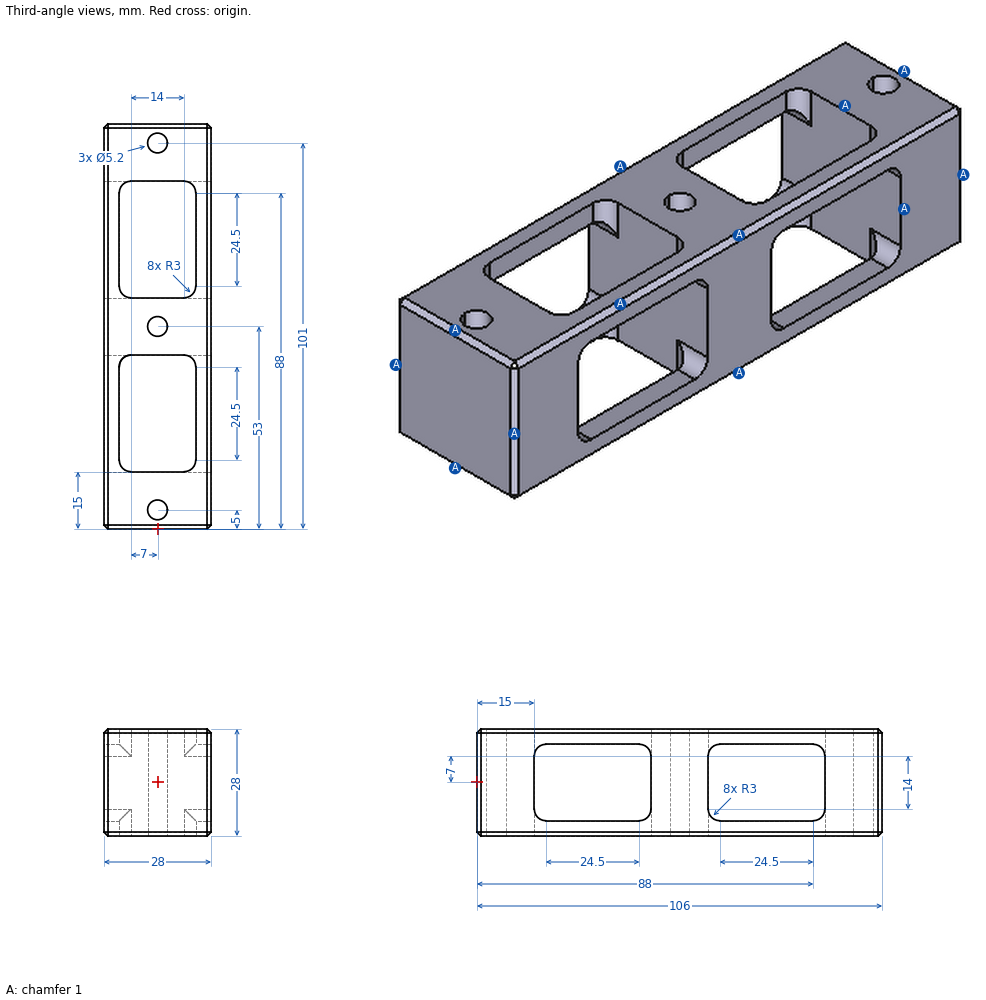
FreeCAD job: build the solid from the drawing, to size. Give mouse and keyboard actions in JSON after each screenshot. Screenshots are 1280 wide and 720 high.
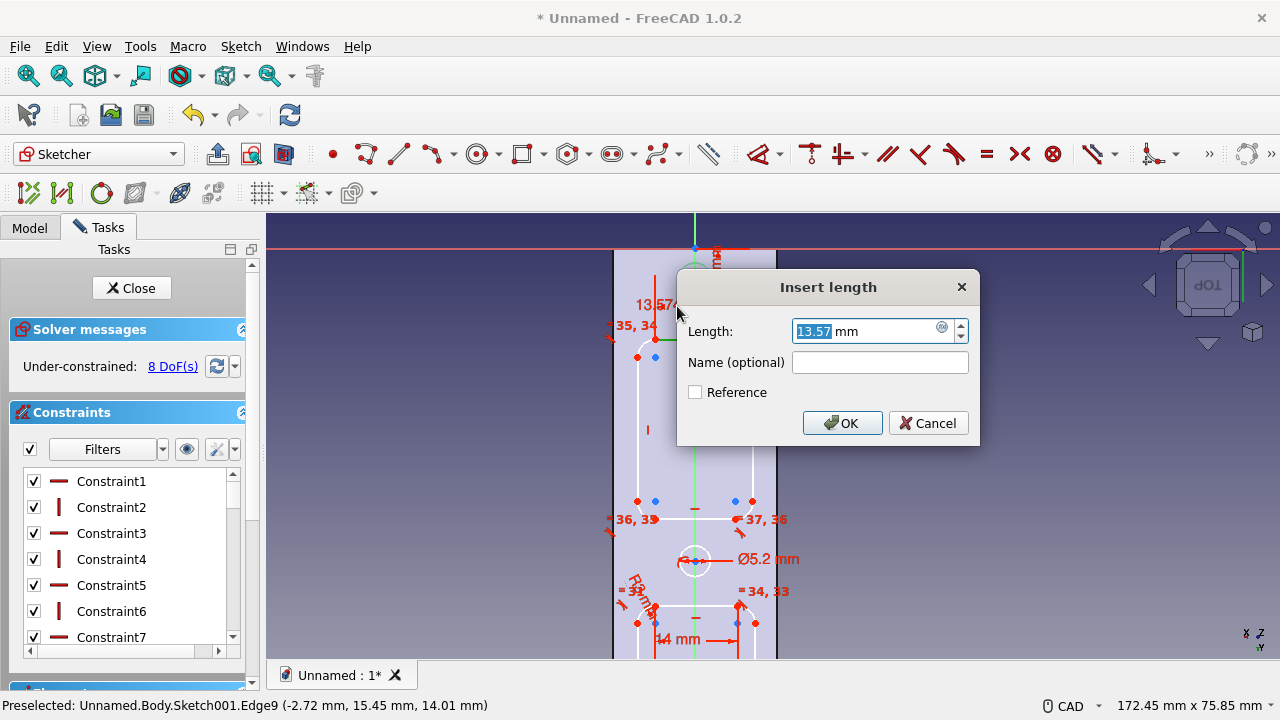
{"action": "type", "text": "14"}
{"action": "key", "text": "Return"}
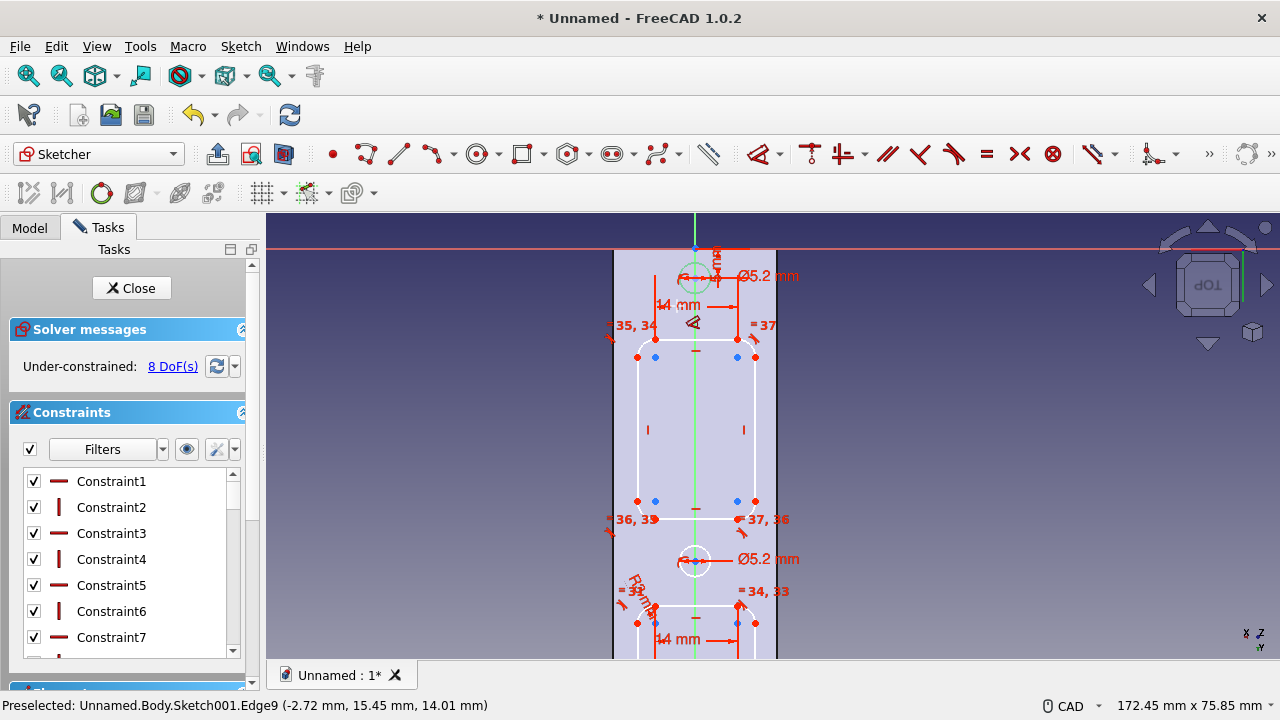
{"action": "left_click", "coordinate": [738, 606]}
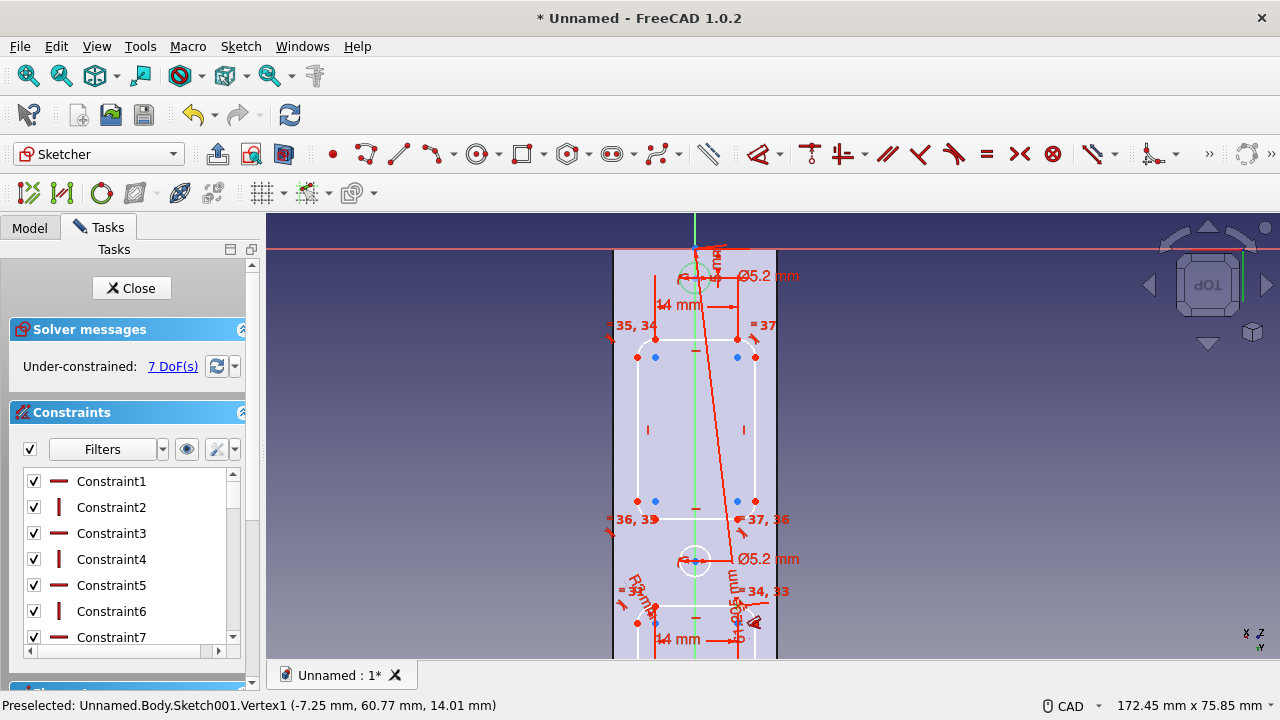
{"action": "key", "text": "Escape"}
{"action": "key", "text": "Escape"}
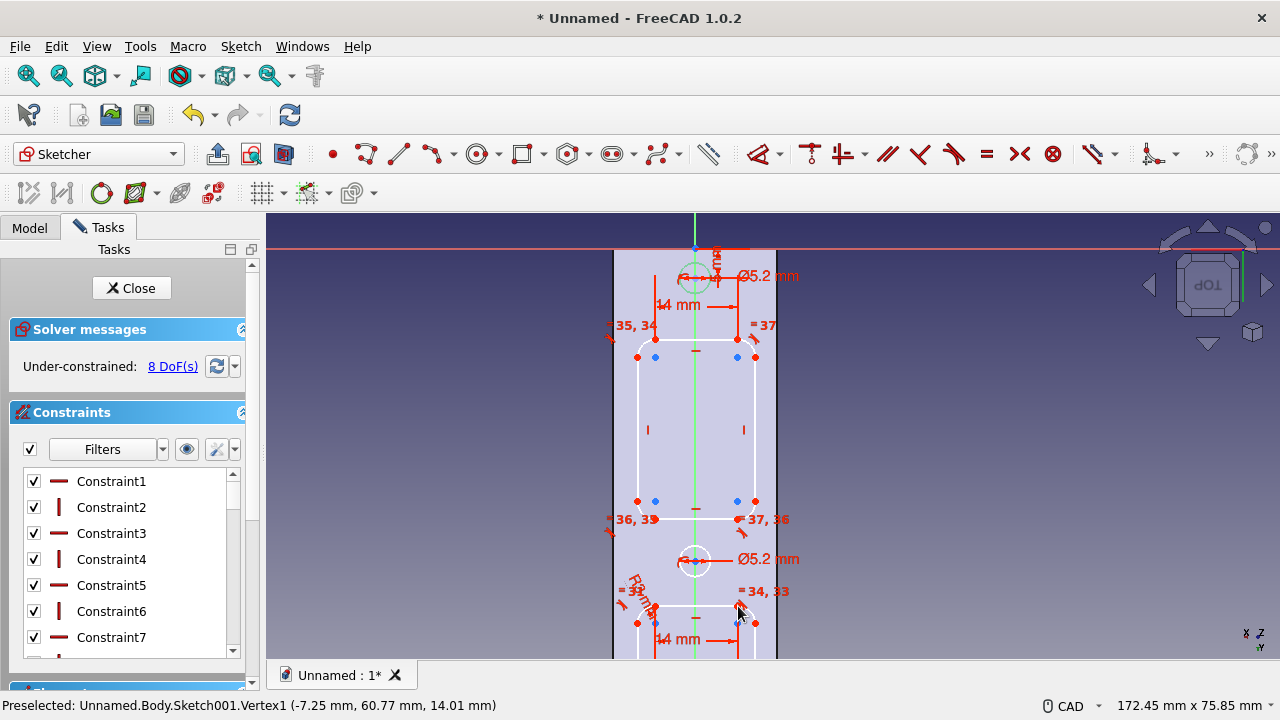
{"action": "left_click", "coordinate": [738, 606]}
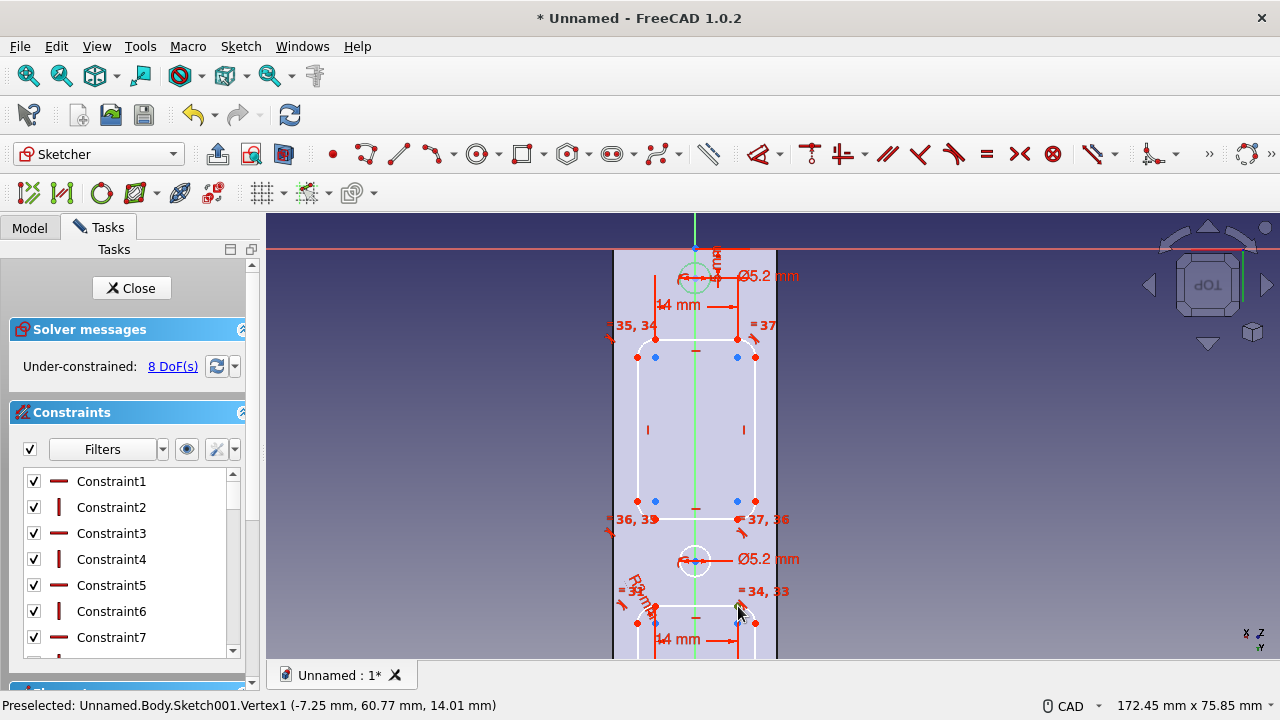
{"action": "left_click", "coordinate": [780, 154]}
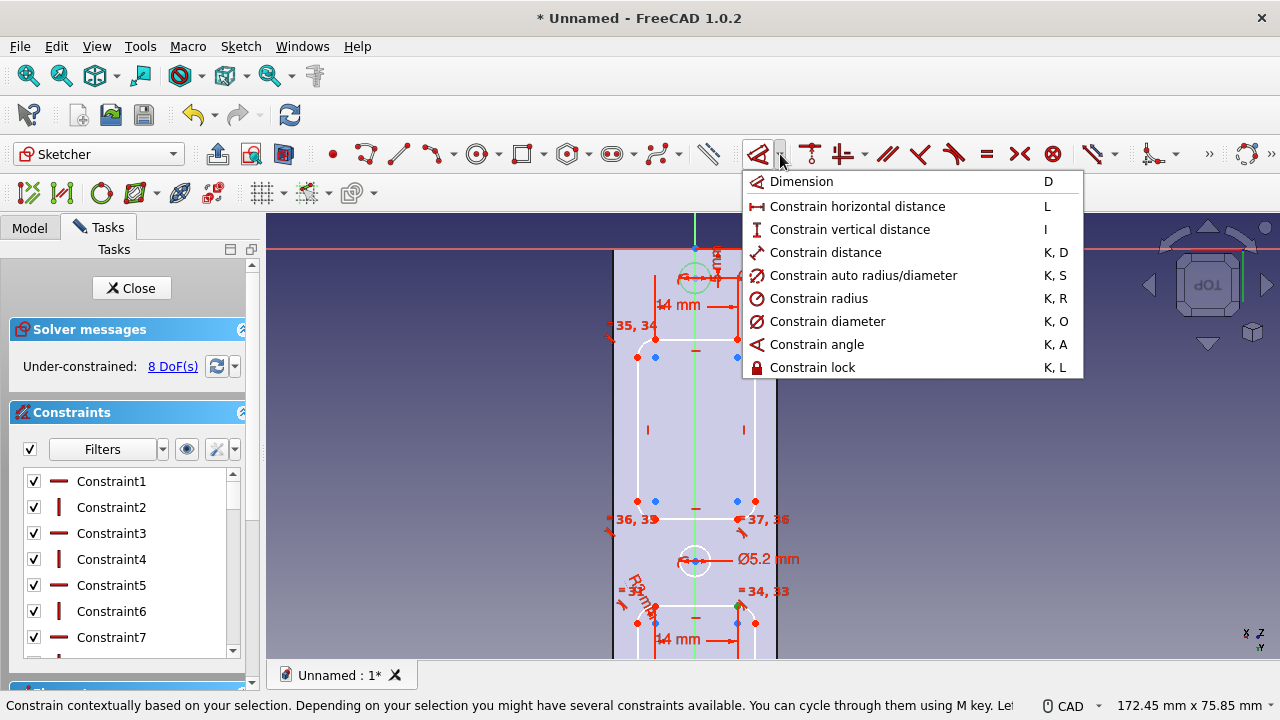
{"action": "left_click", "coordinate": [913, 206]}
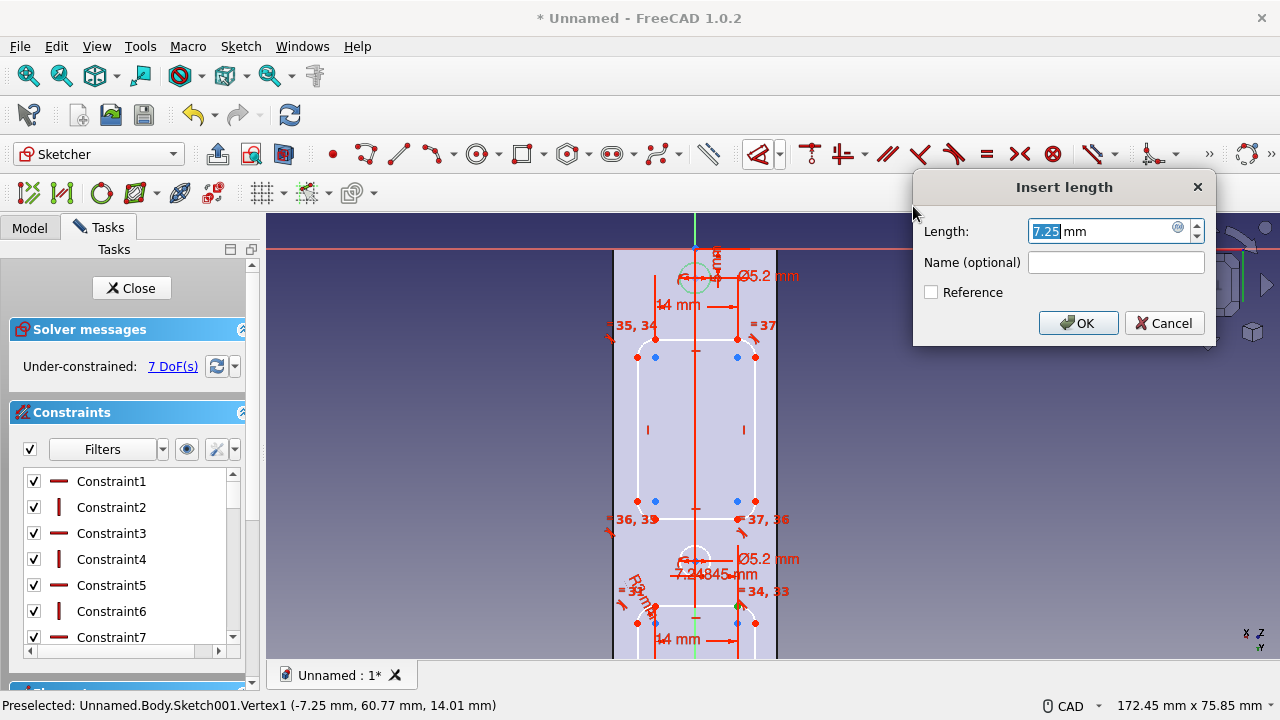
{"action": "type", "text": "7"}
{"action": "key", "text": "Return"}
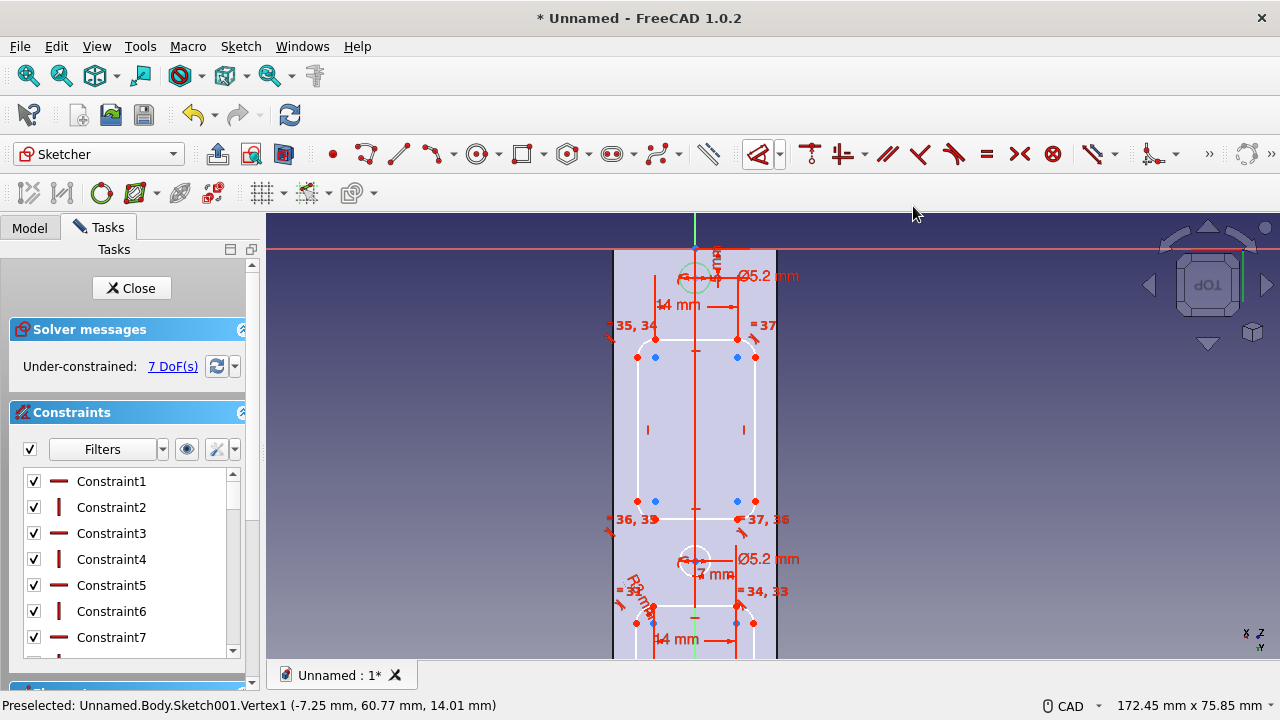
{"action": "left_click", "coordinate": [738, 340]}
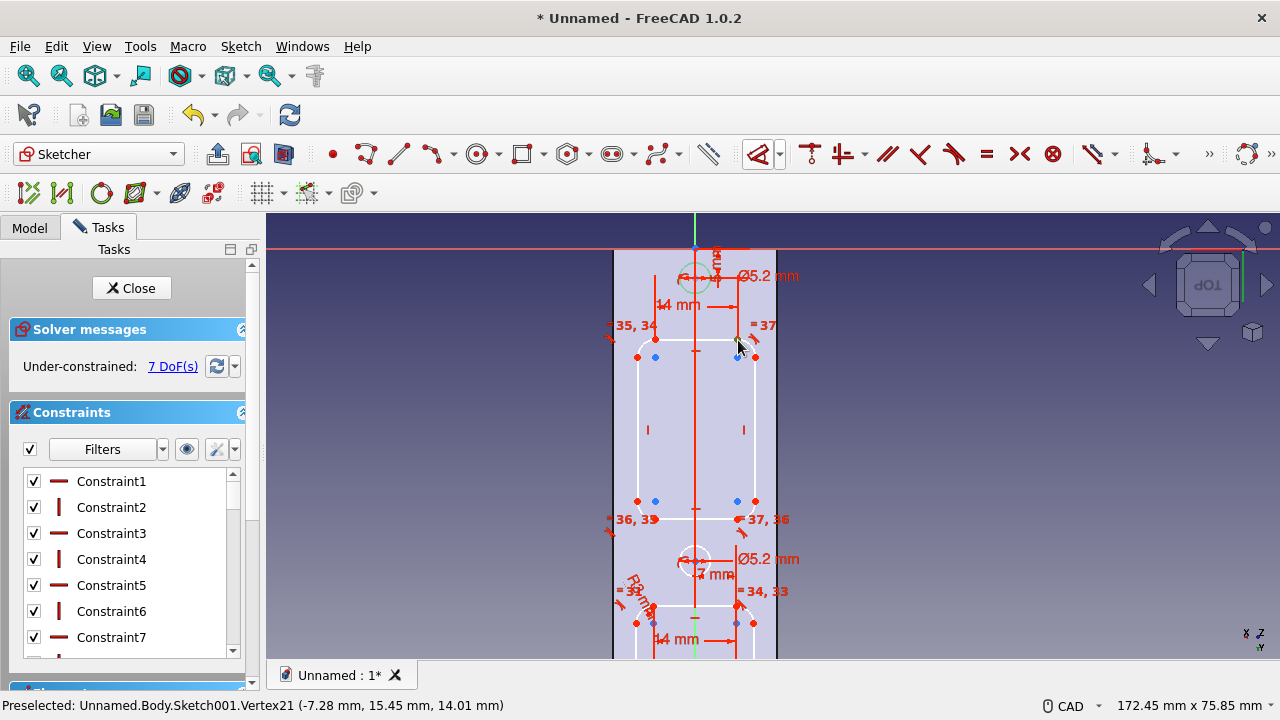
{"action": "left_click", "coordinate": [780, 154]}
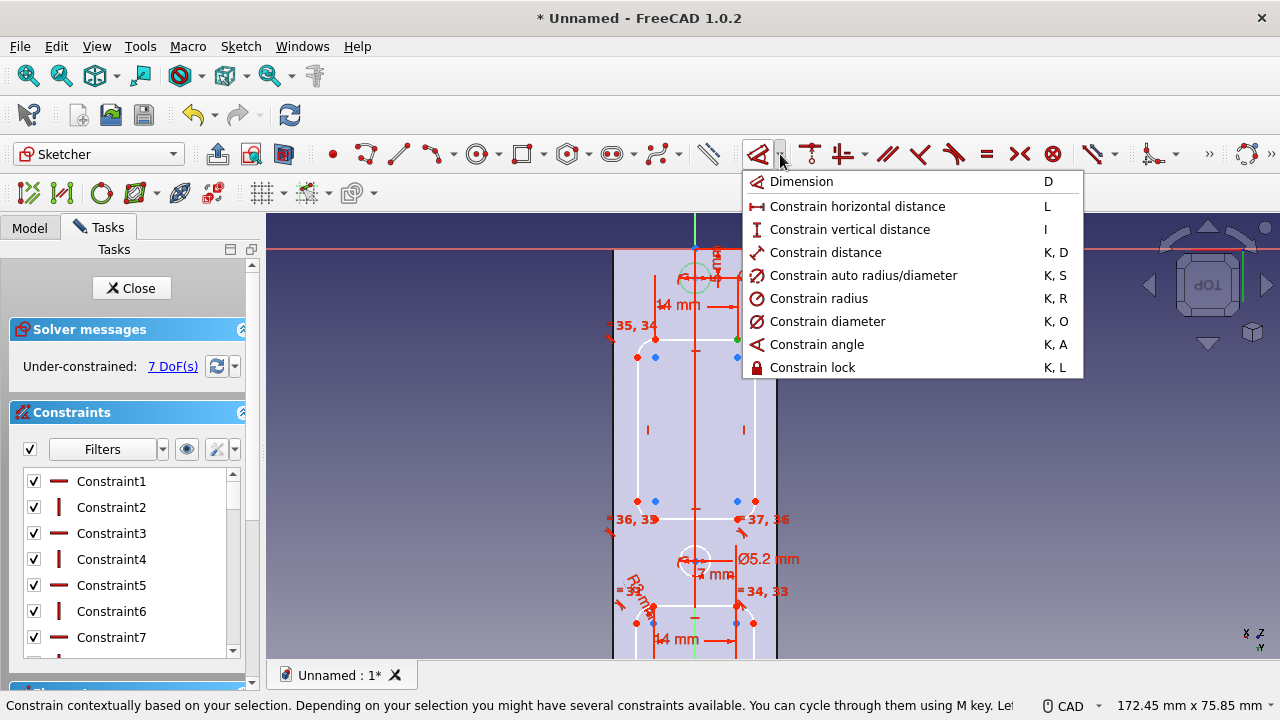
{"action": "left_click", "coordinate": [913, 206]}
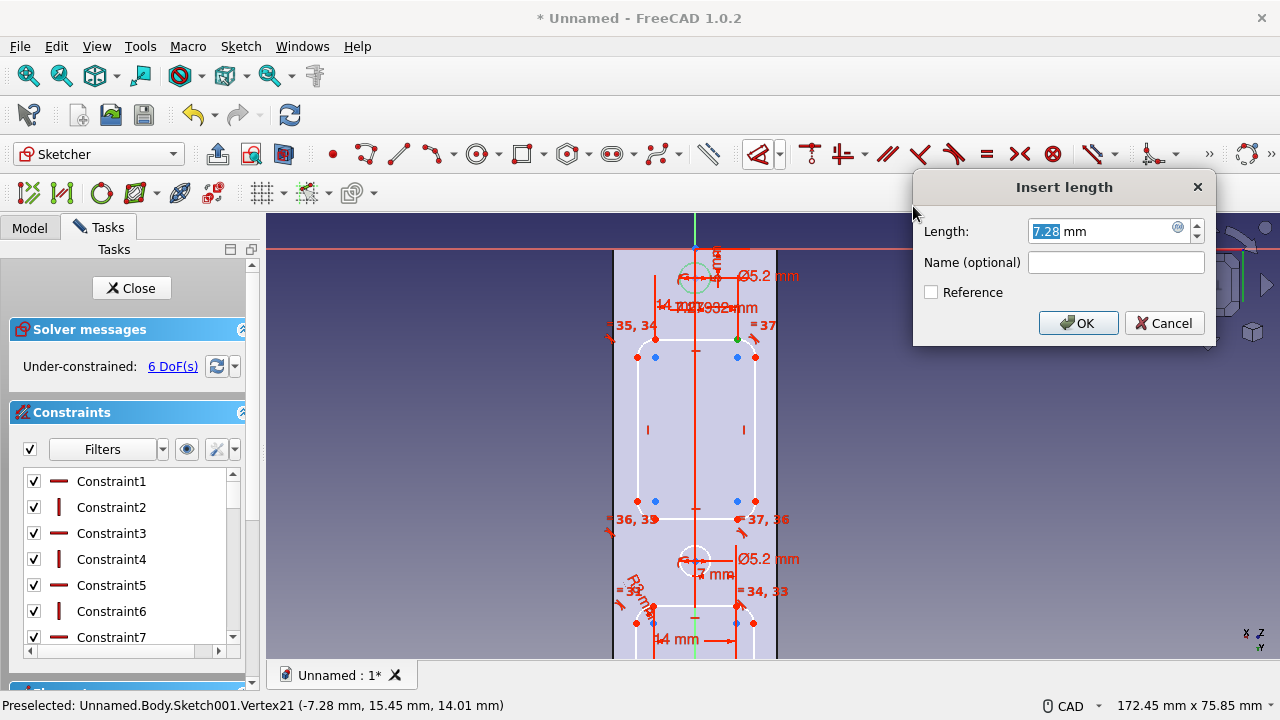
{"action": "type", "text": "7"}
{"action": "key", "text": "Return"}